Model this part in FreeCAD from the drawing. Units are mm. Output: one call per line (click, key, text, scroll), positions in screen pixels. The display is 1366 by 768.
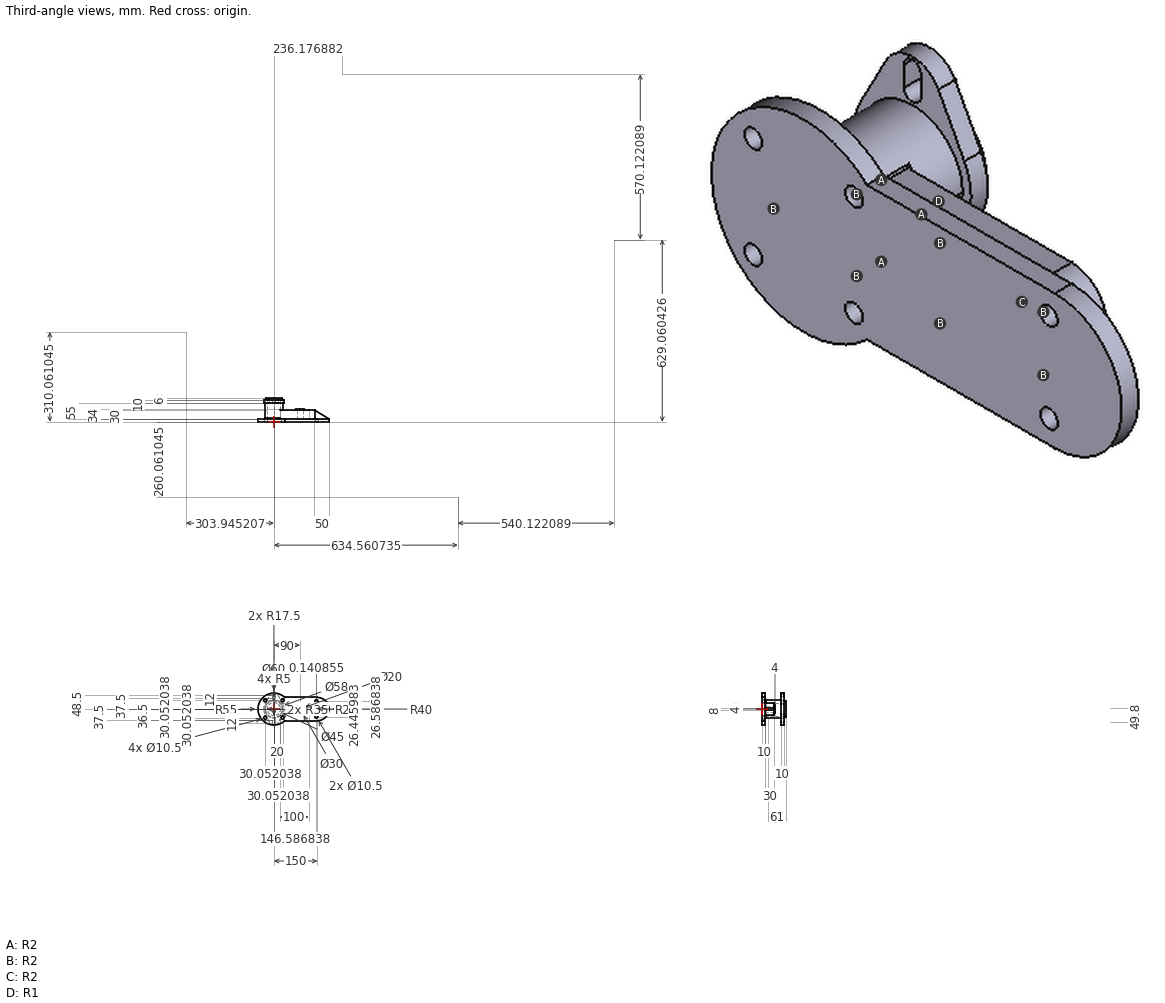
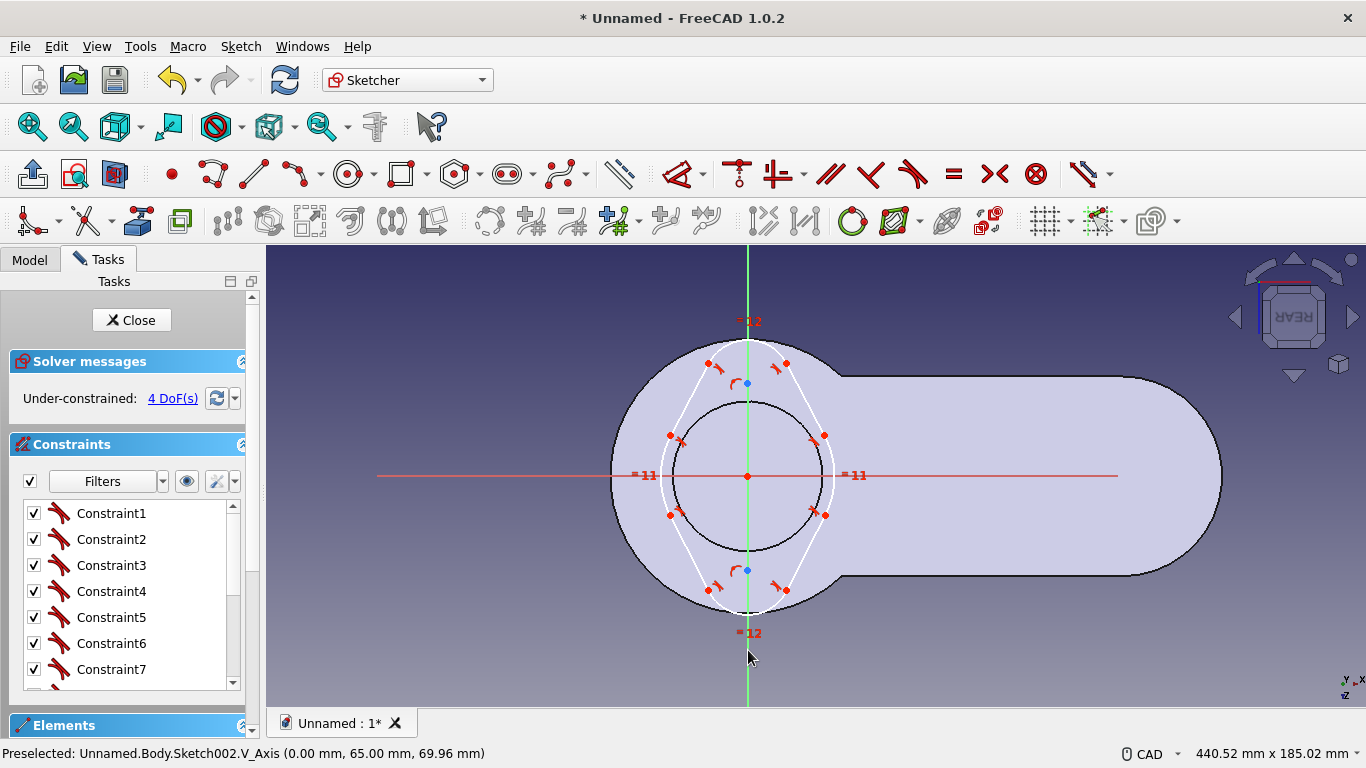
click(676, 174)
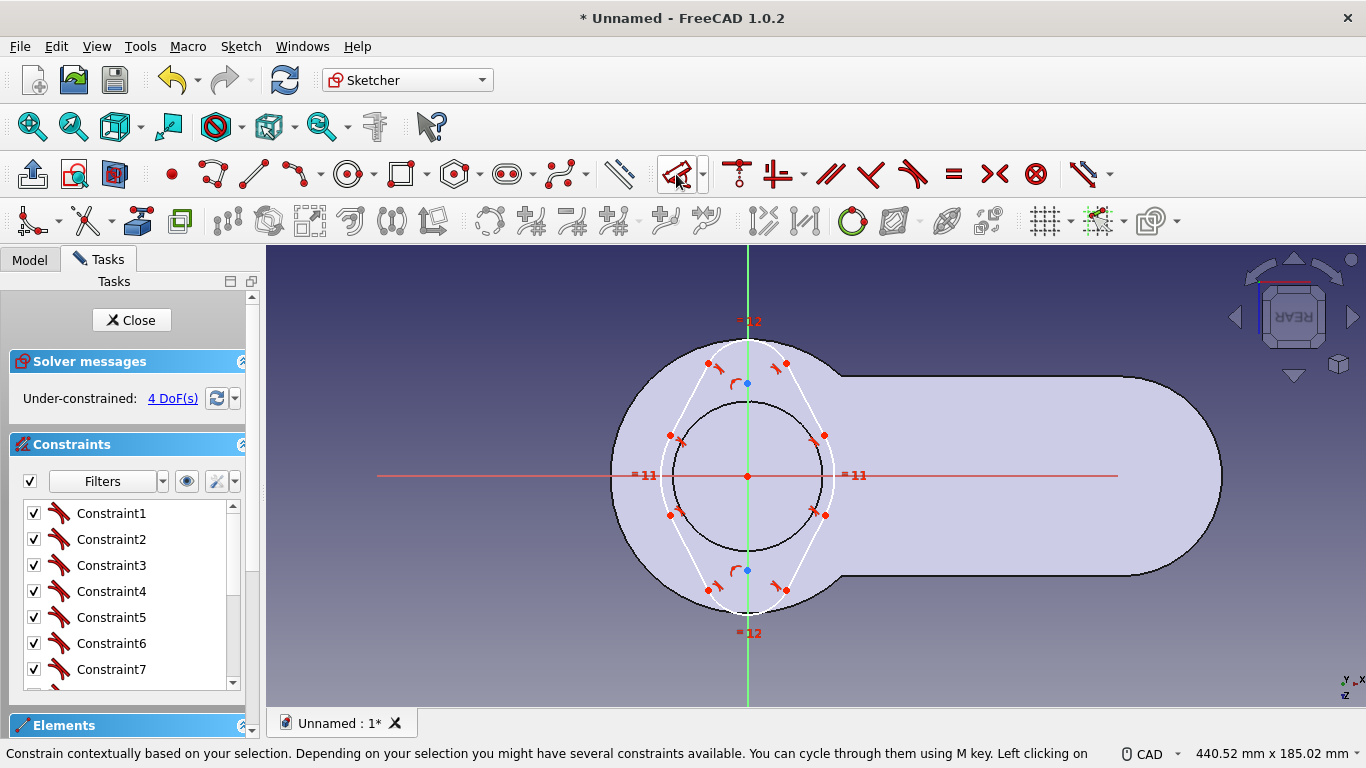
click(663, 459)
click(632, 453)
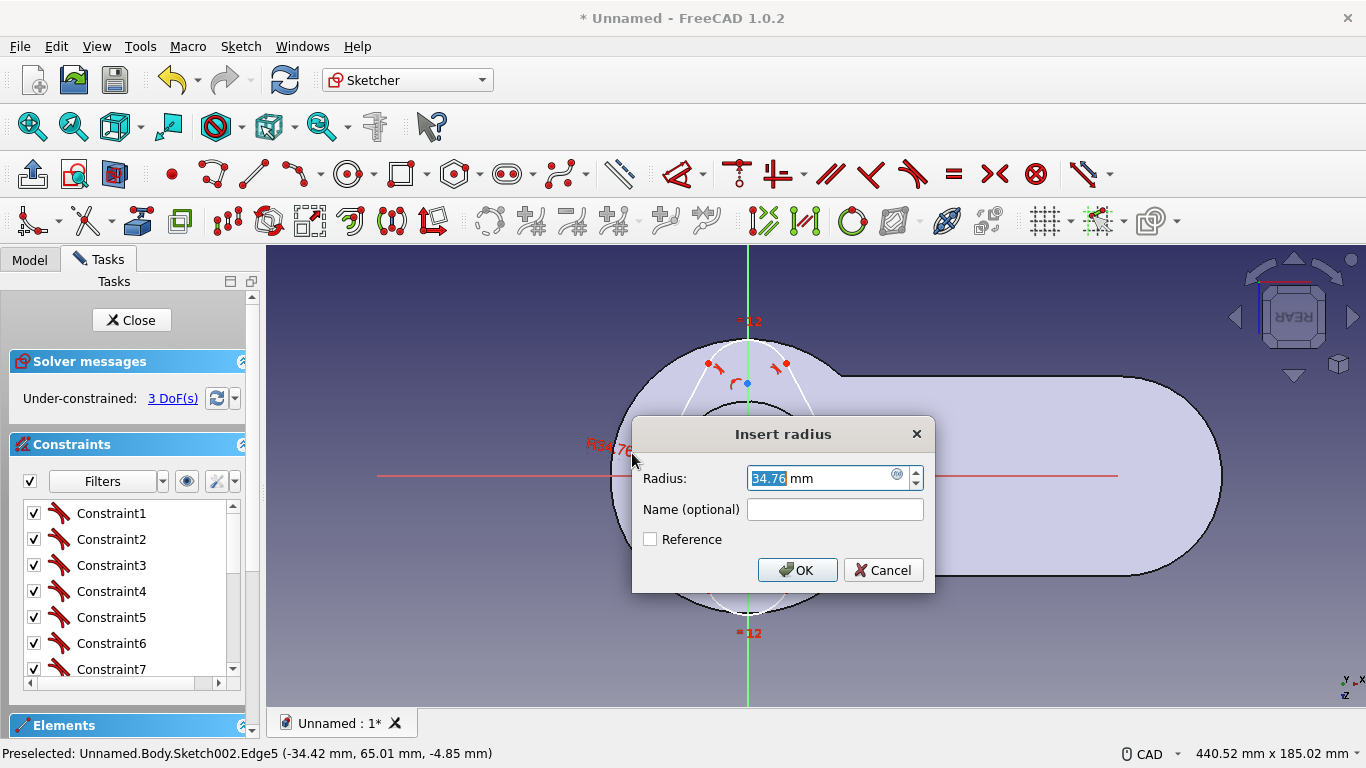
text(35)
key(Return)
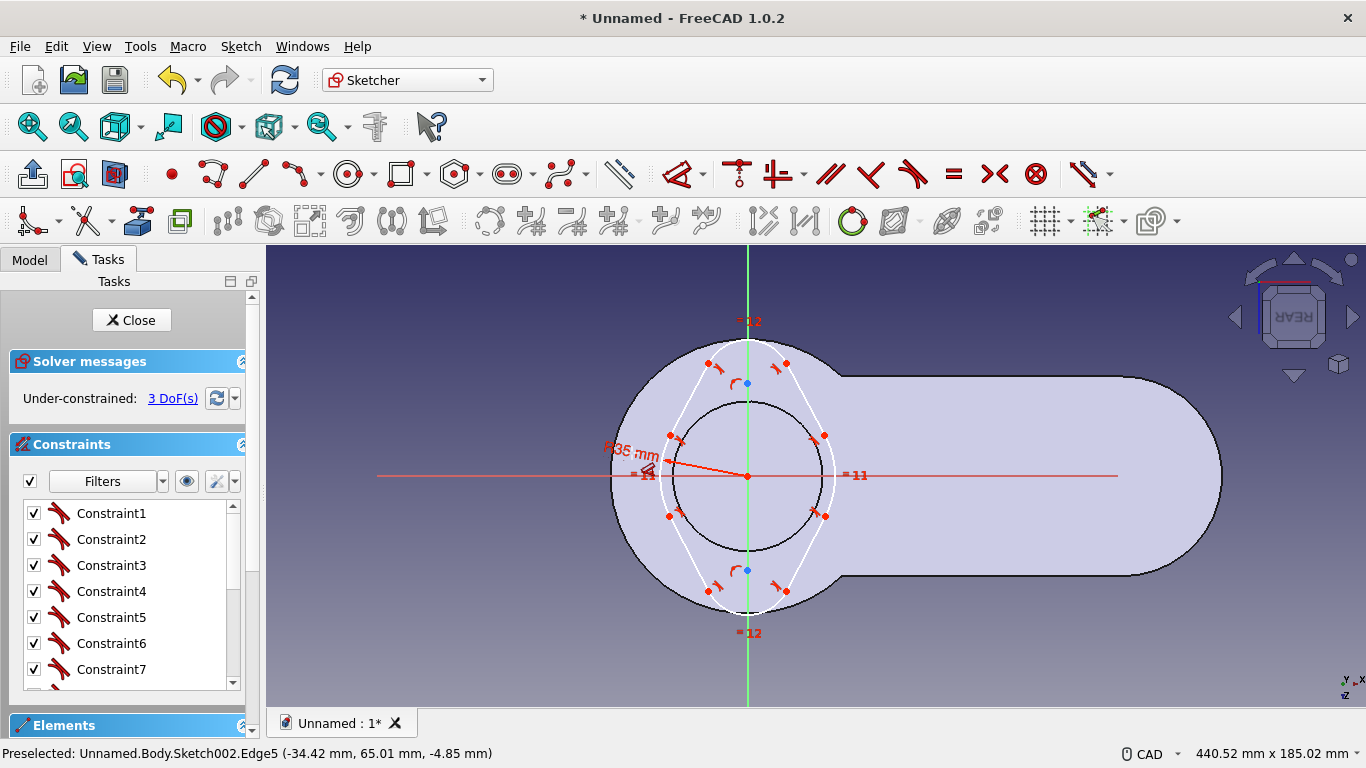
click(729, 611)
click(715, 640)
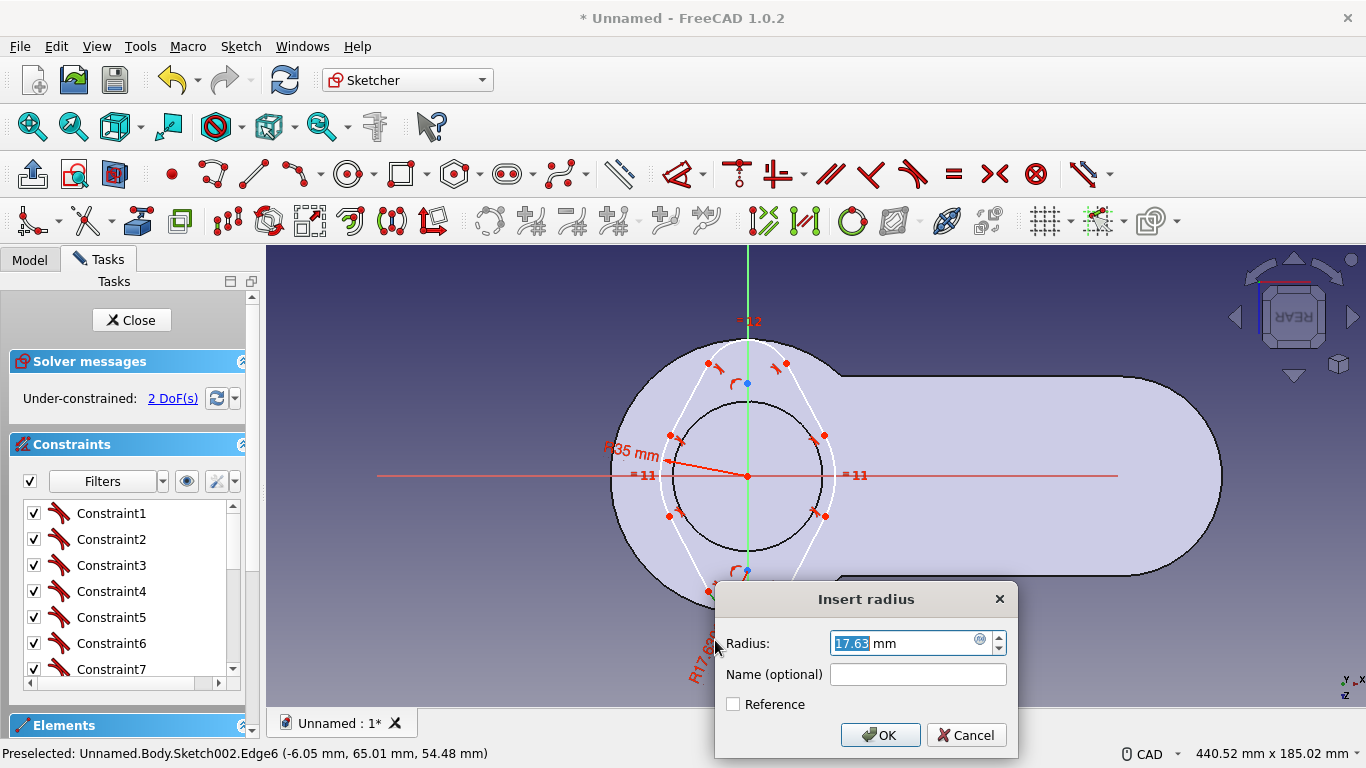
text(17.5)
key(Return)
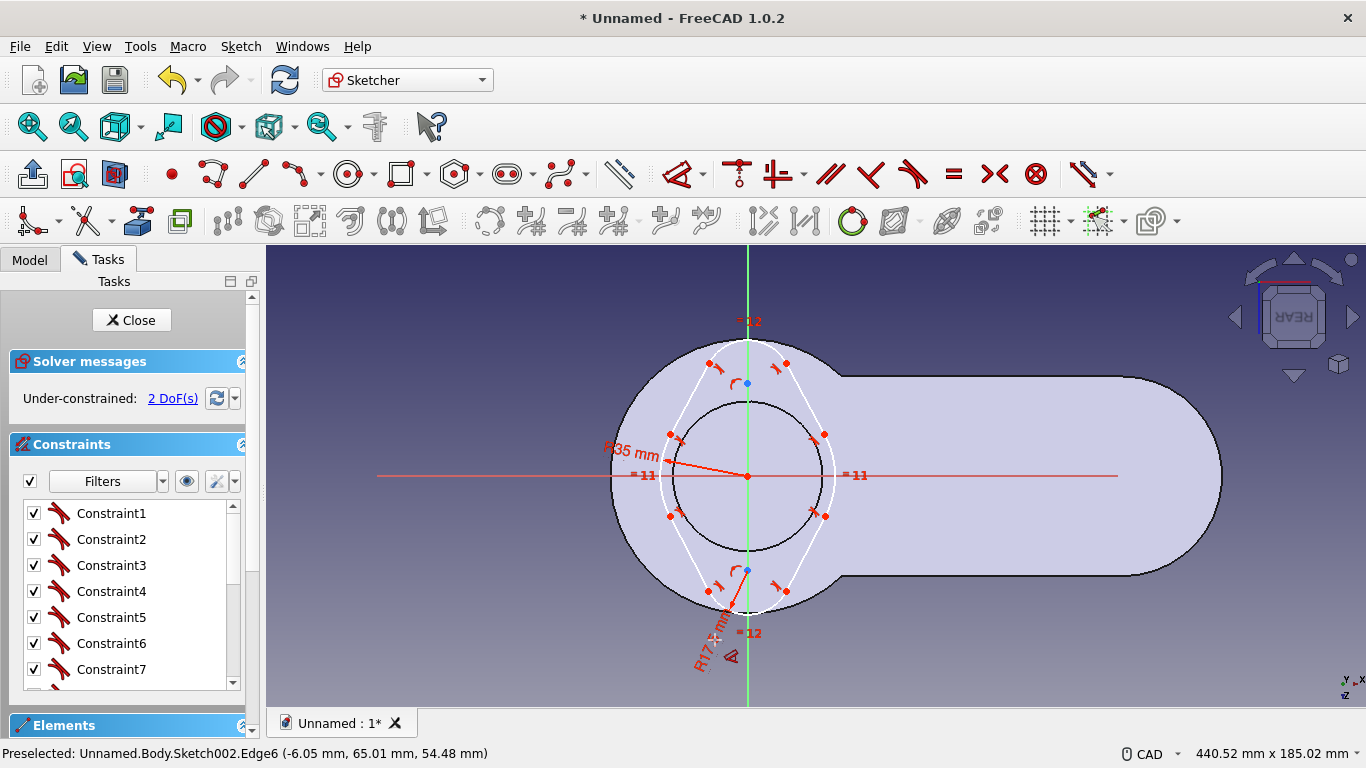
click(748, 571)
click(782, 524)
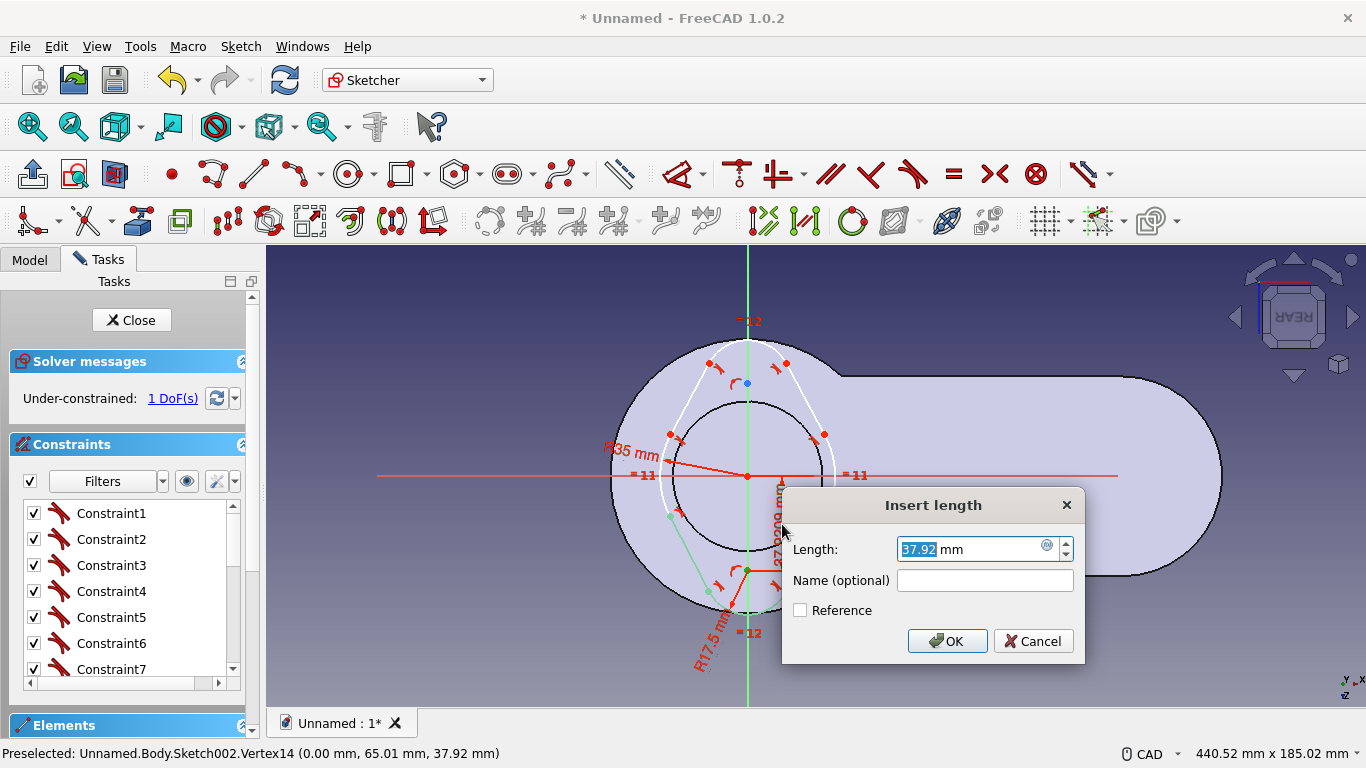
text(37.5)
key(Return)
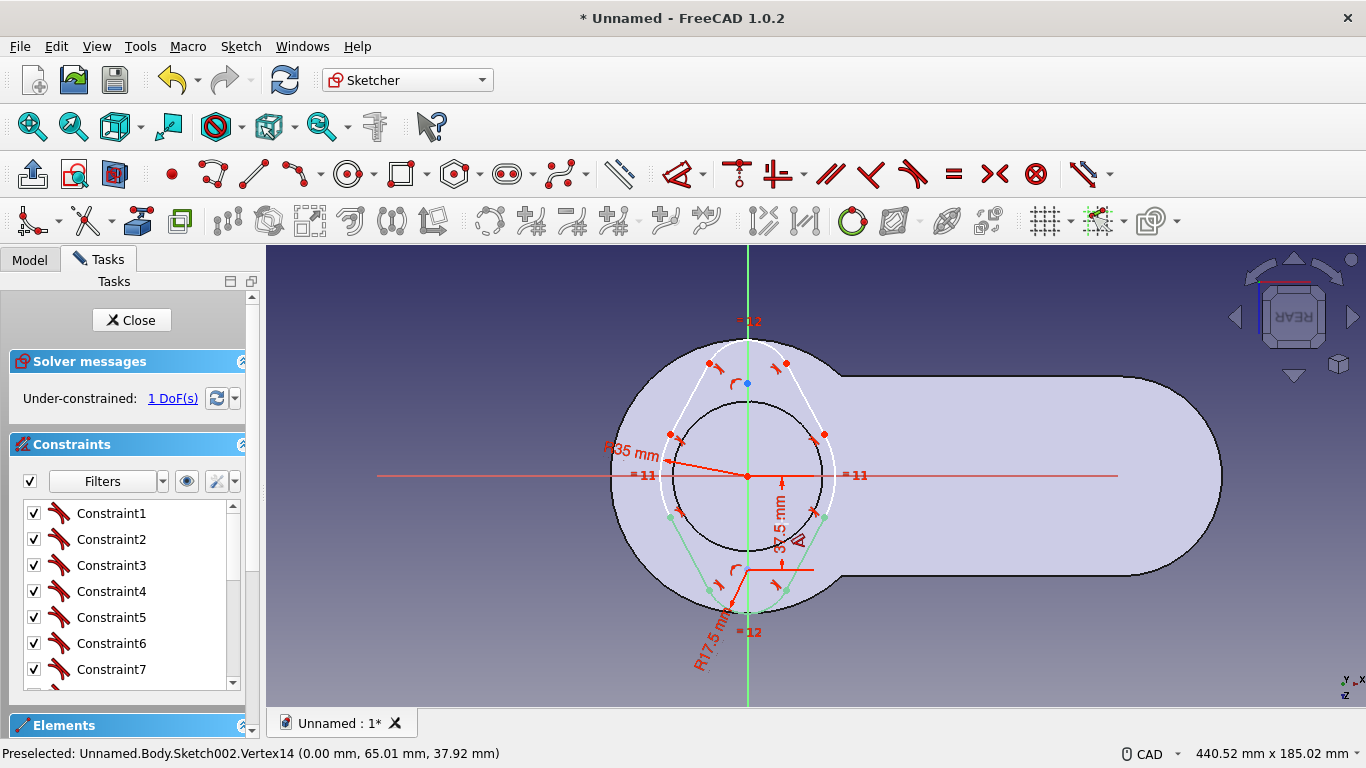
click(748, 384)
click(782, 430)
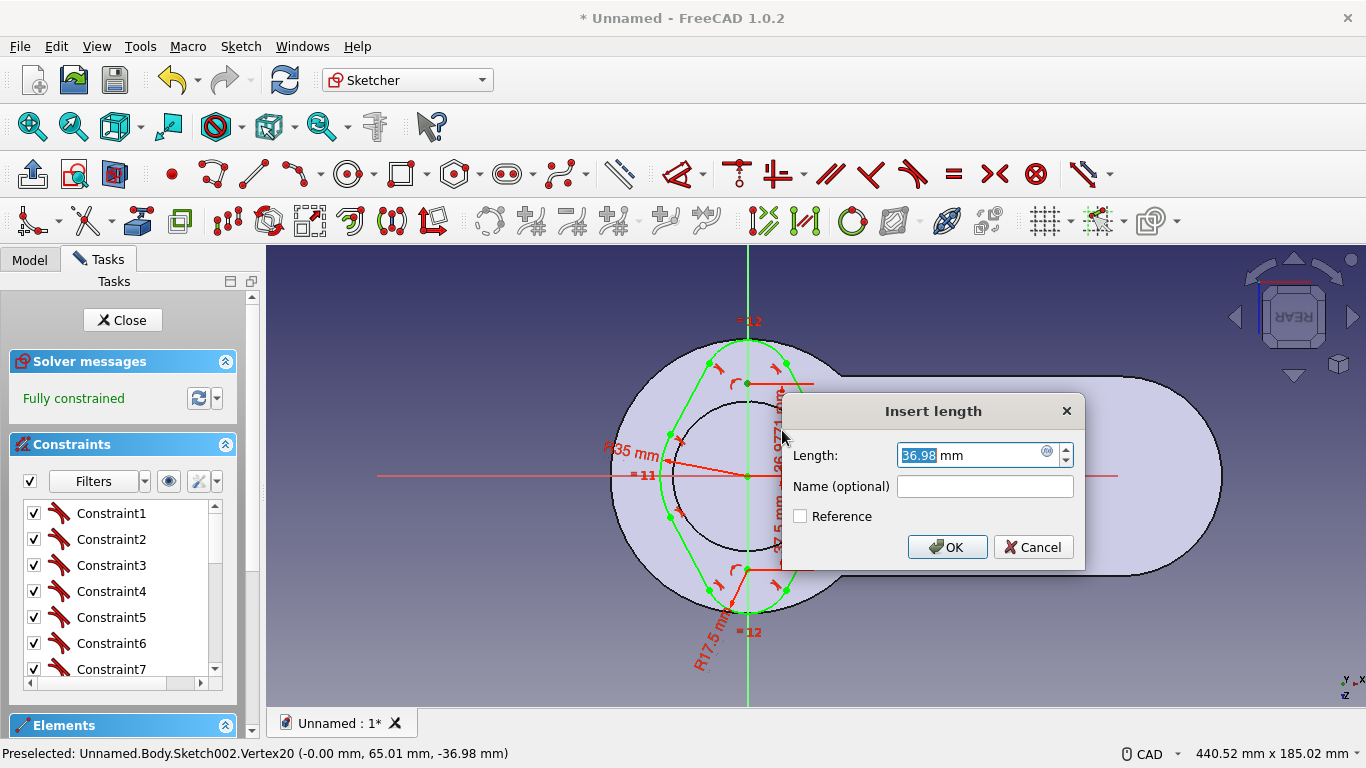
text(37.5)
key(Return)
key(Escape)